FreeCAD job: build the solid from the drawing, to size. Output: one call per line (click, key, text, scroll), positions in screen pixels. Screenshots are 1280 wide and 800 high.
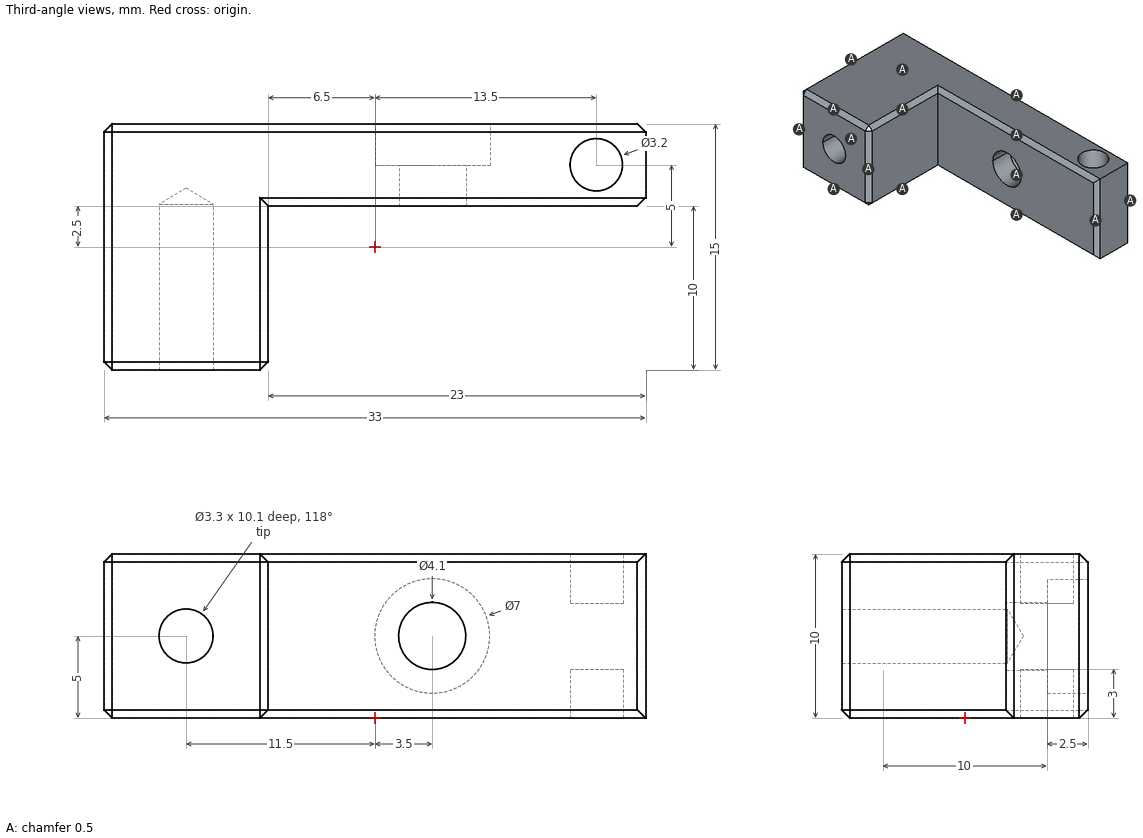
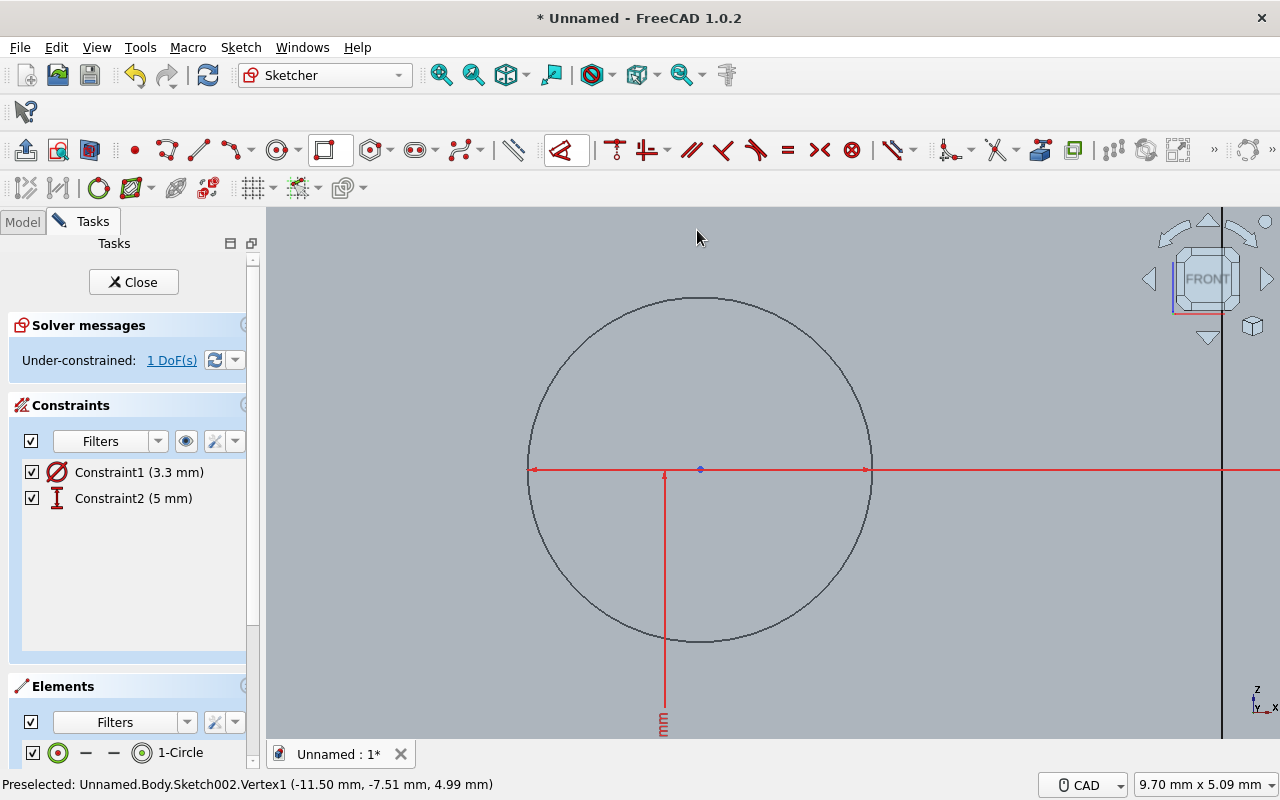
click(700, 470)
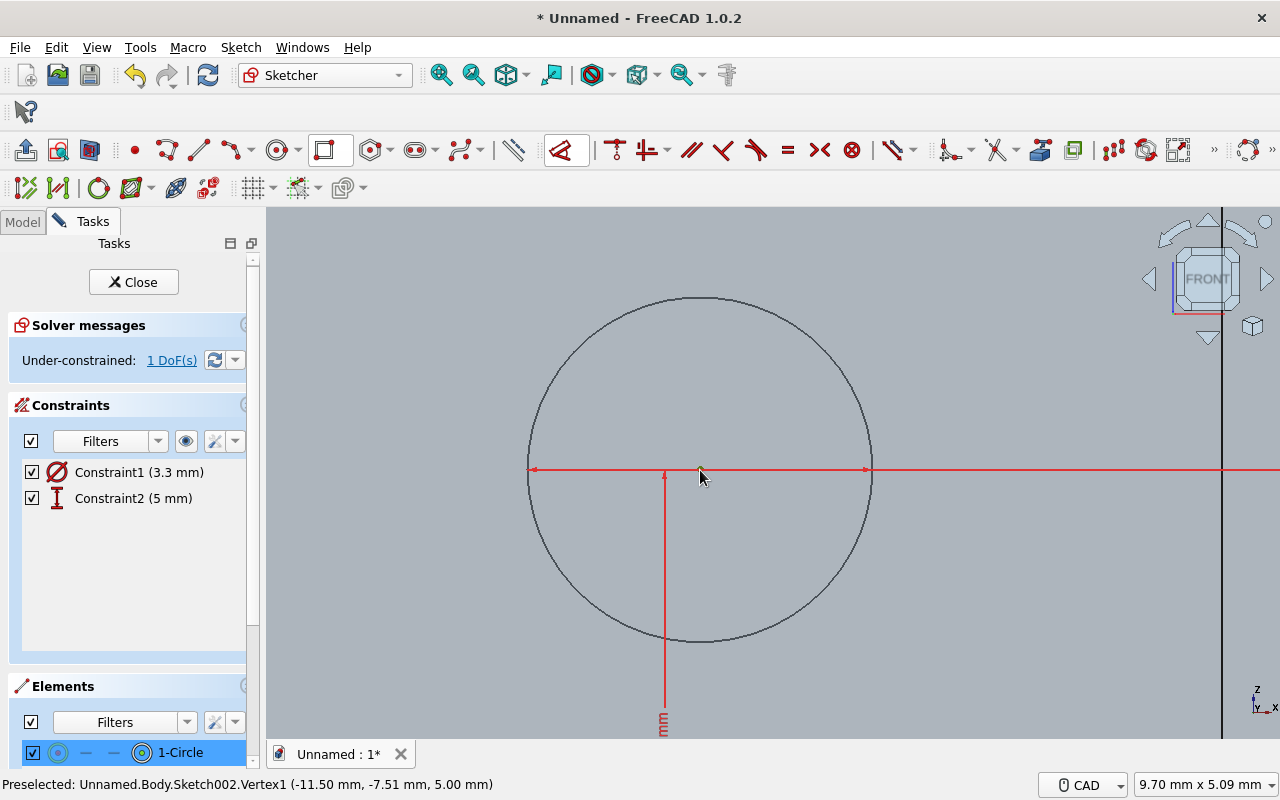
click(584, 150)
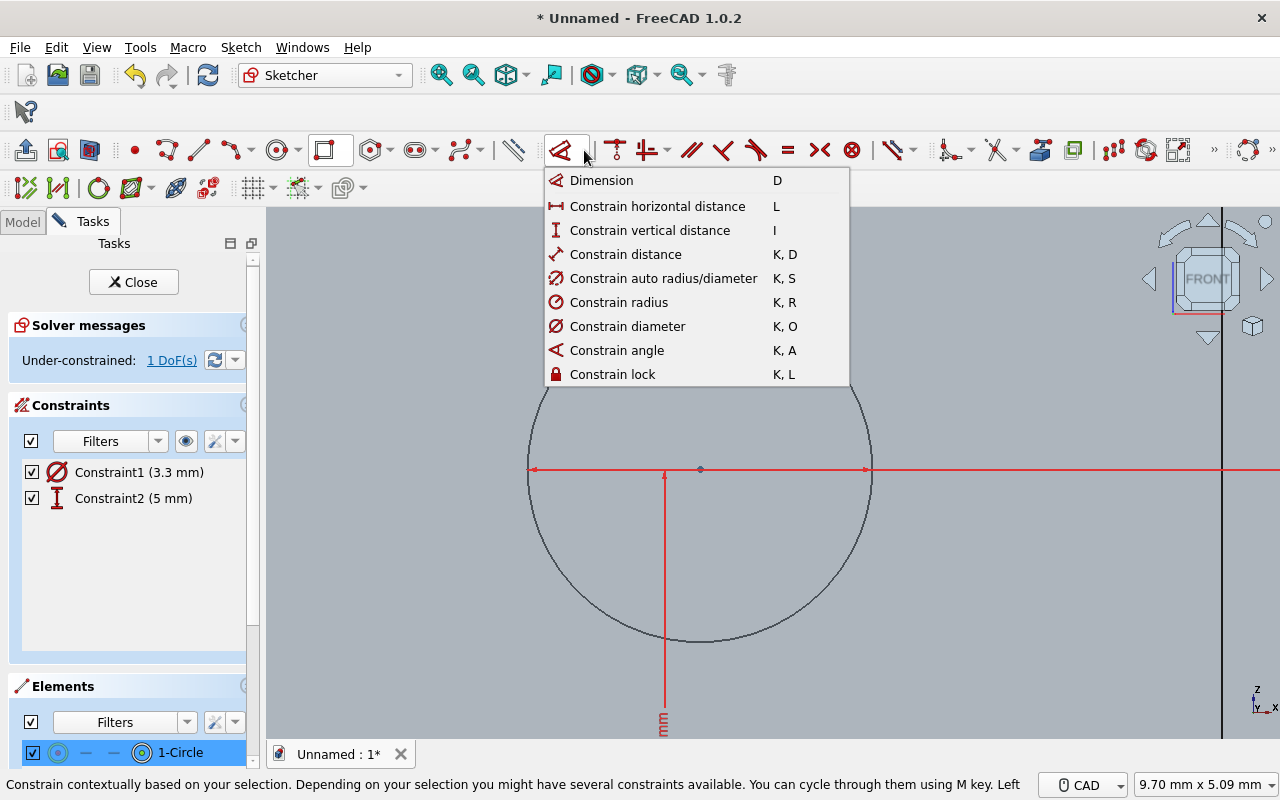
click(697, 206)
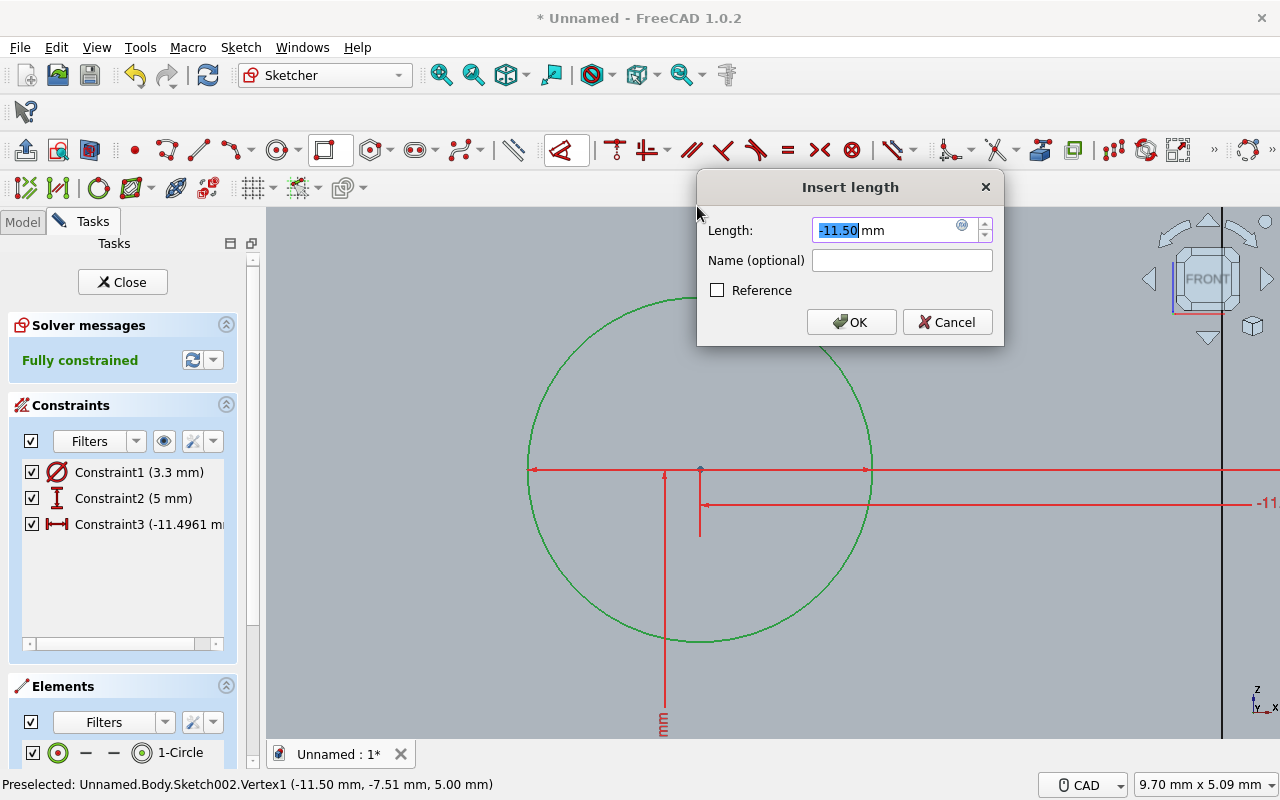
text(-11.5)
key(Return)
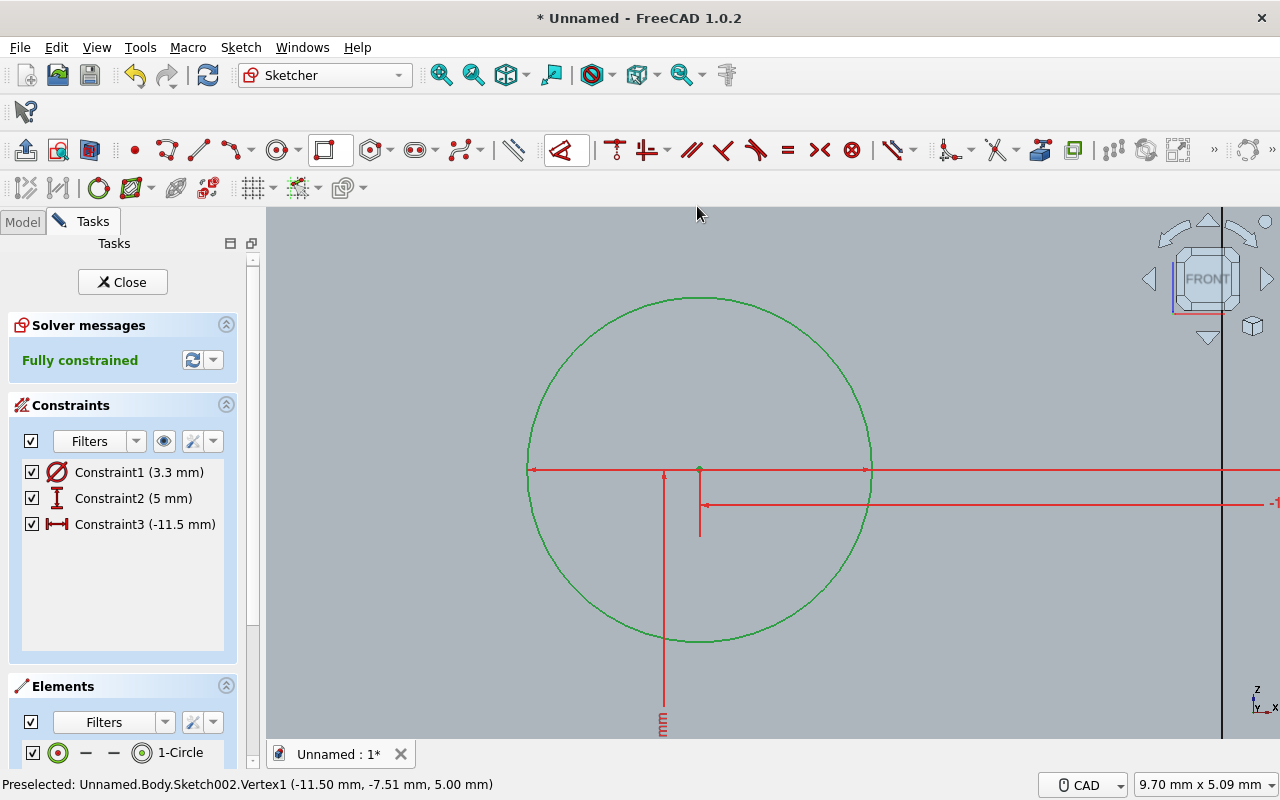
click(123, 282)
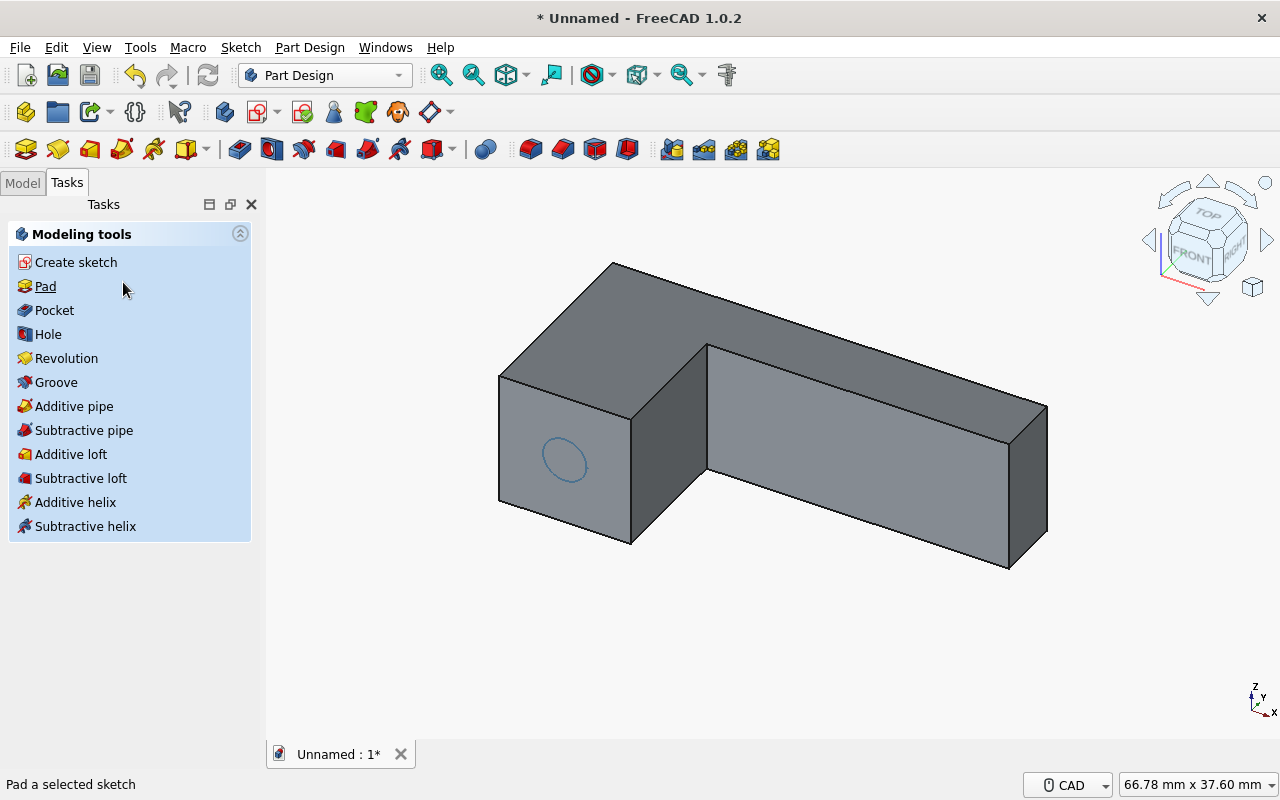
click(272, 150)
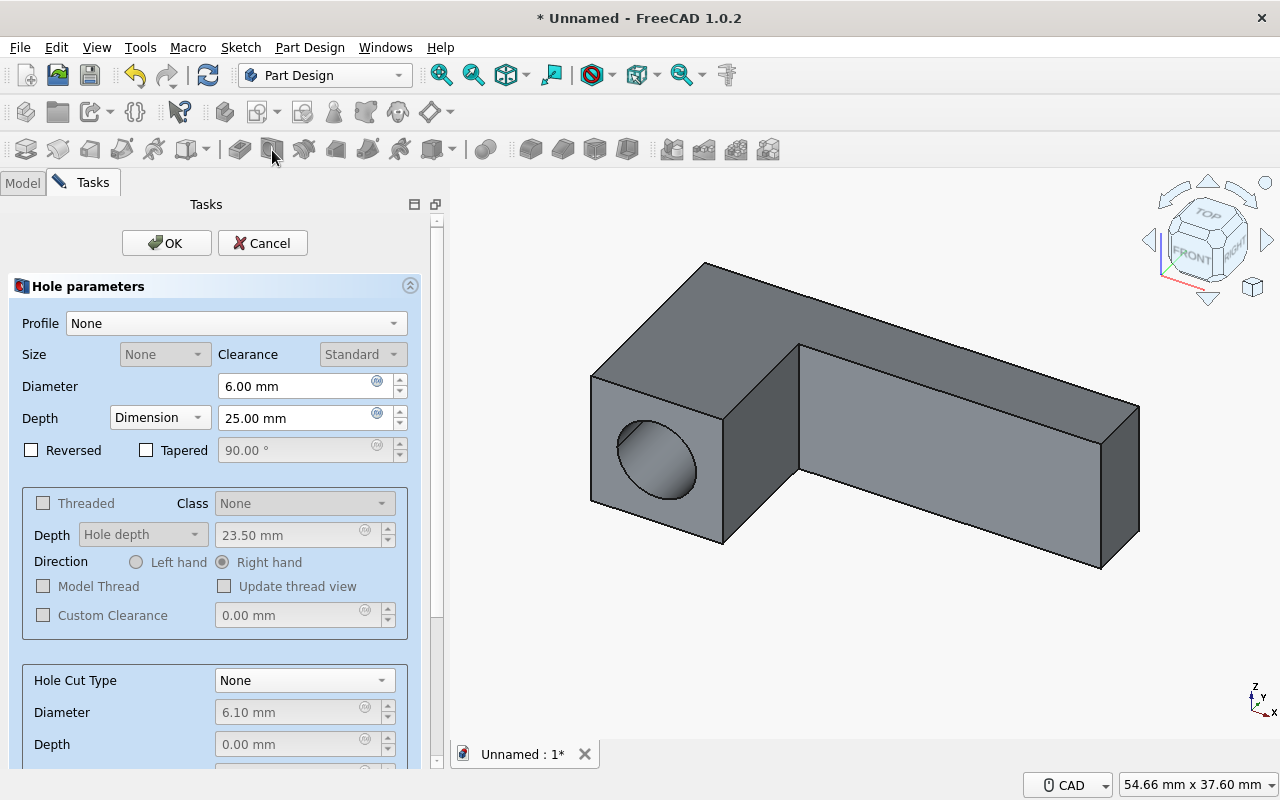
triple_click(305, 386)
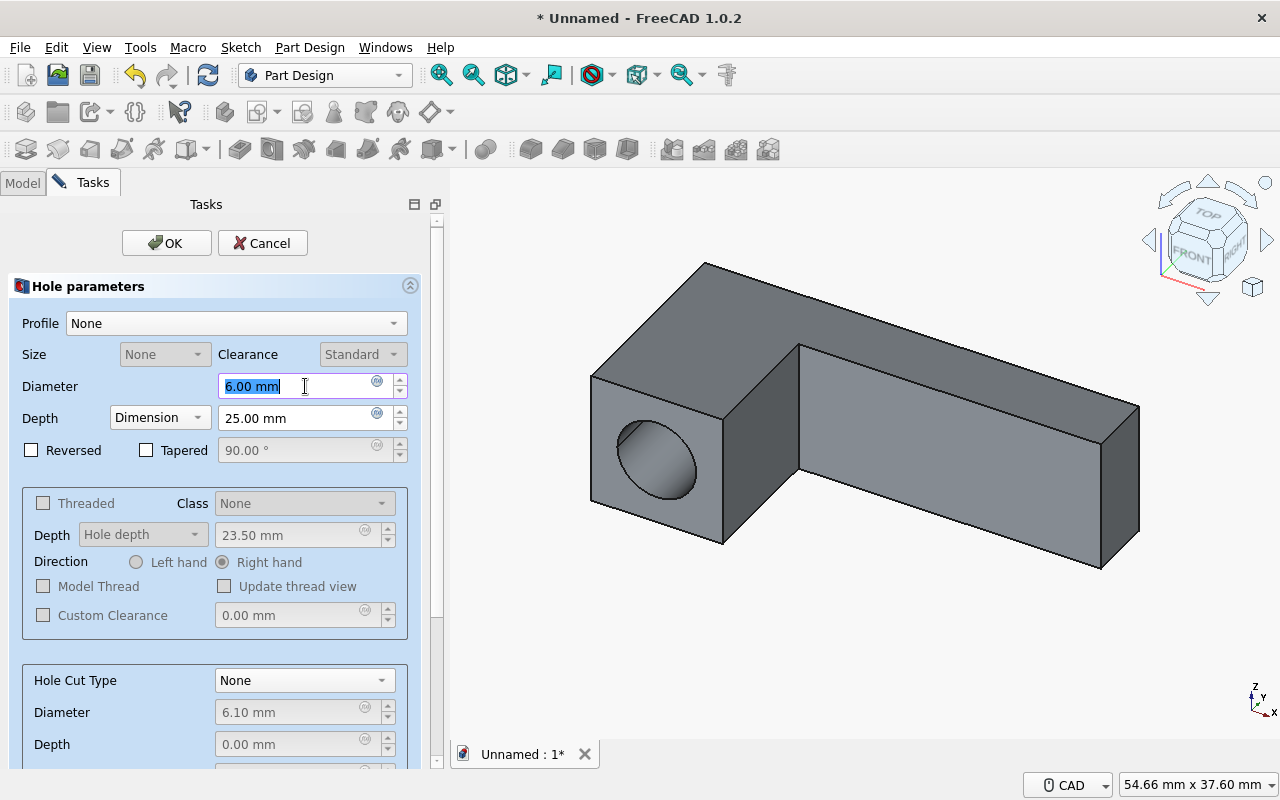
text(3.3)
key(Tab)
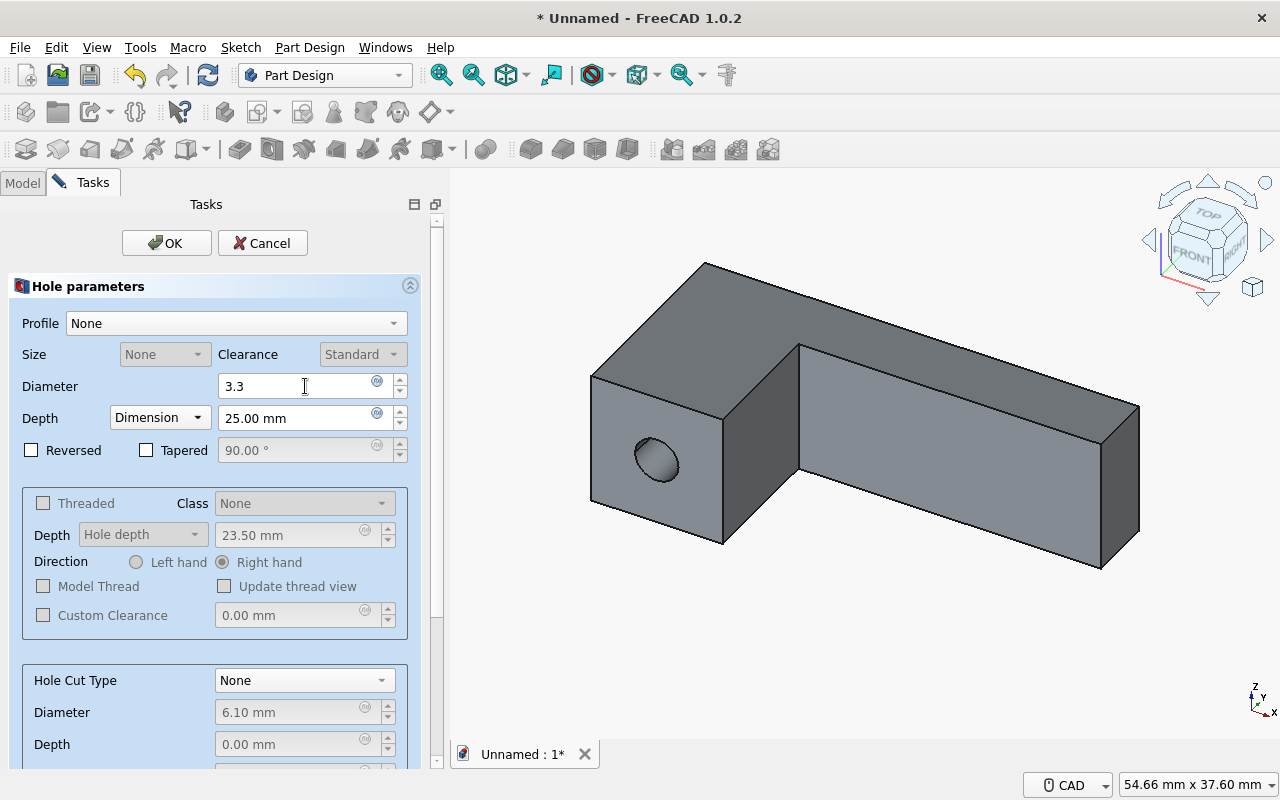
triple_click(305, 418)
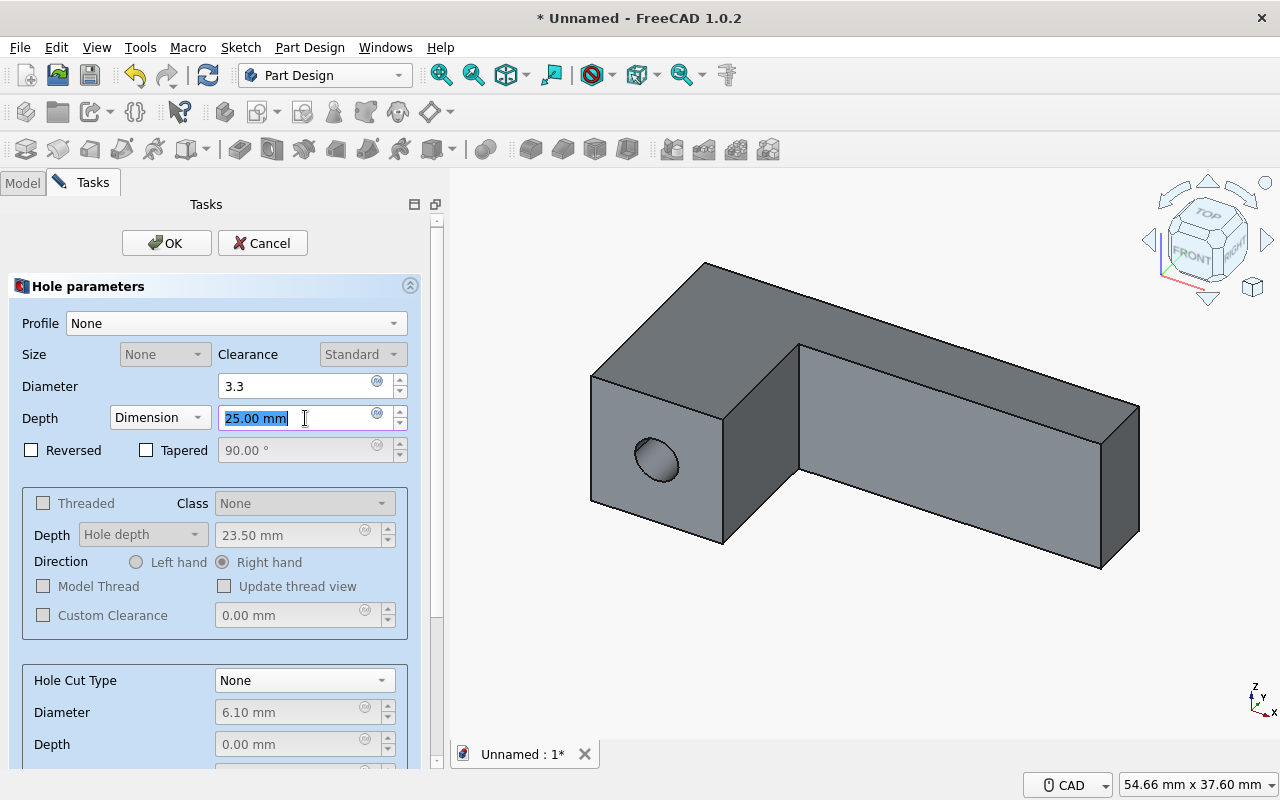
text(10.1)
key(Tab)